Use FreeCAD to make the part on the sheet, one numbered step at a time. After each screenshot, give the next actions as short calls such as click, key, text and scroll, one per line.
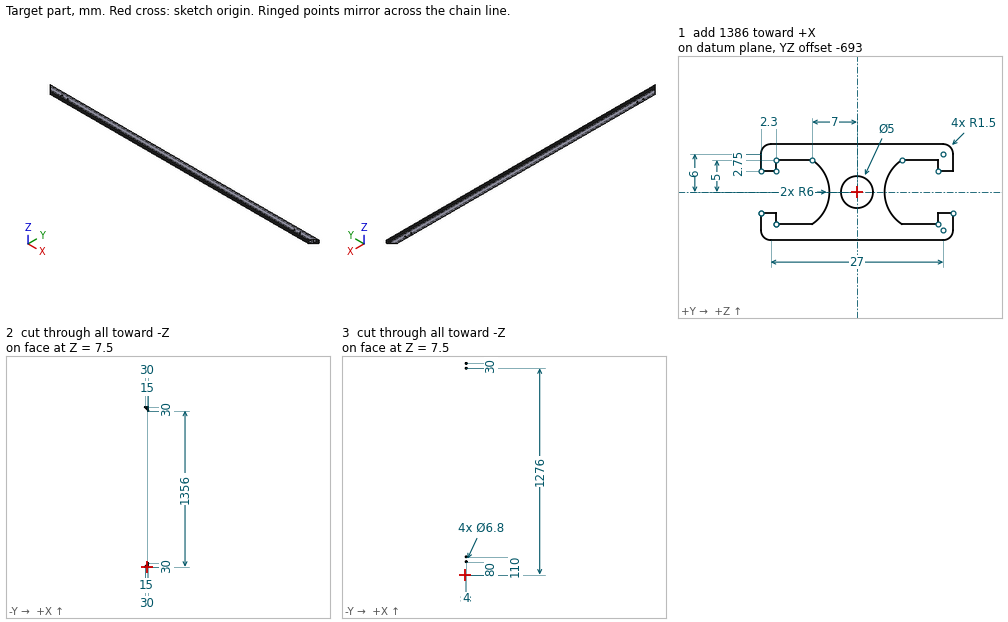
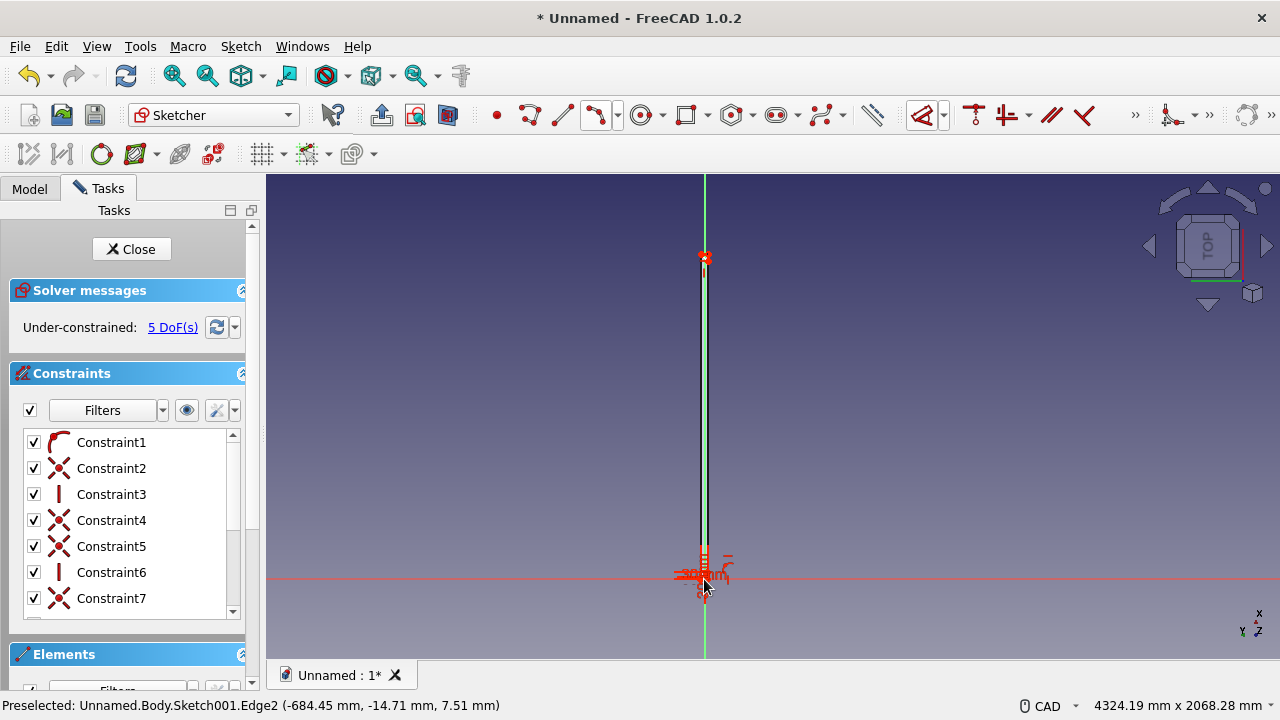
scroll(708, 260, up, 12)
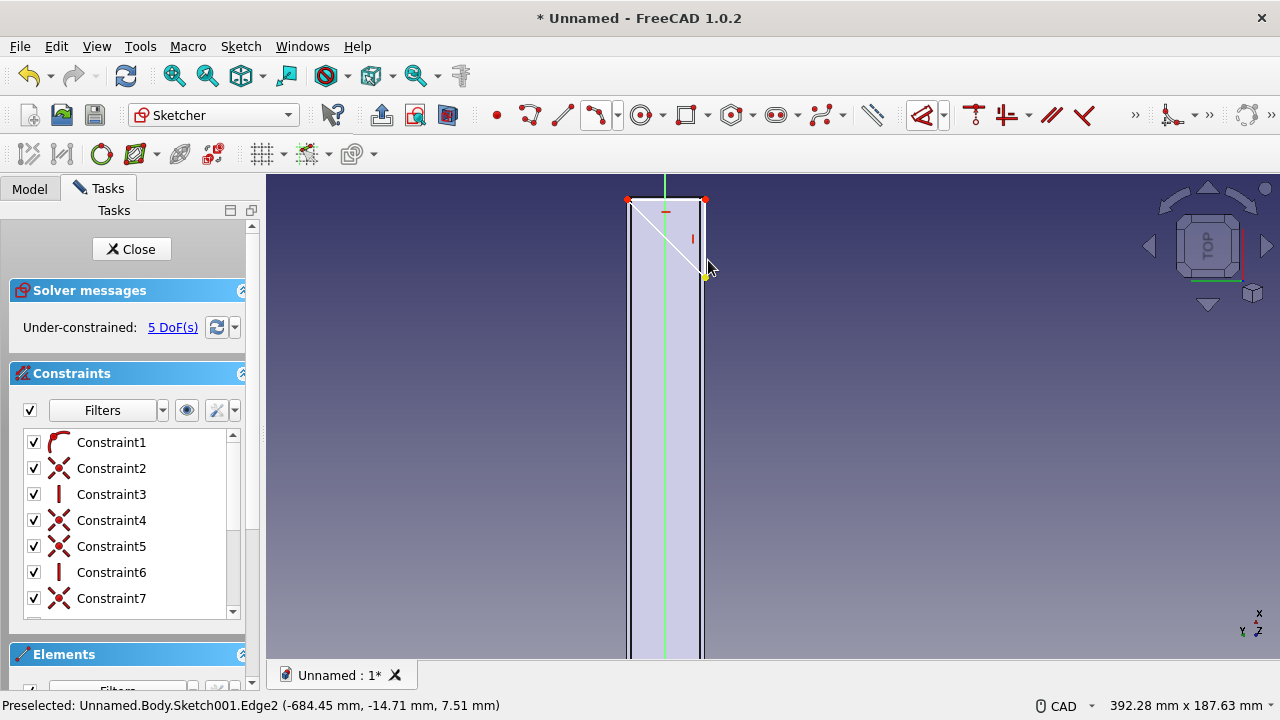
click(705, 254)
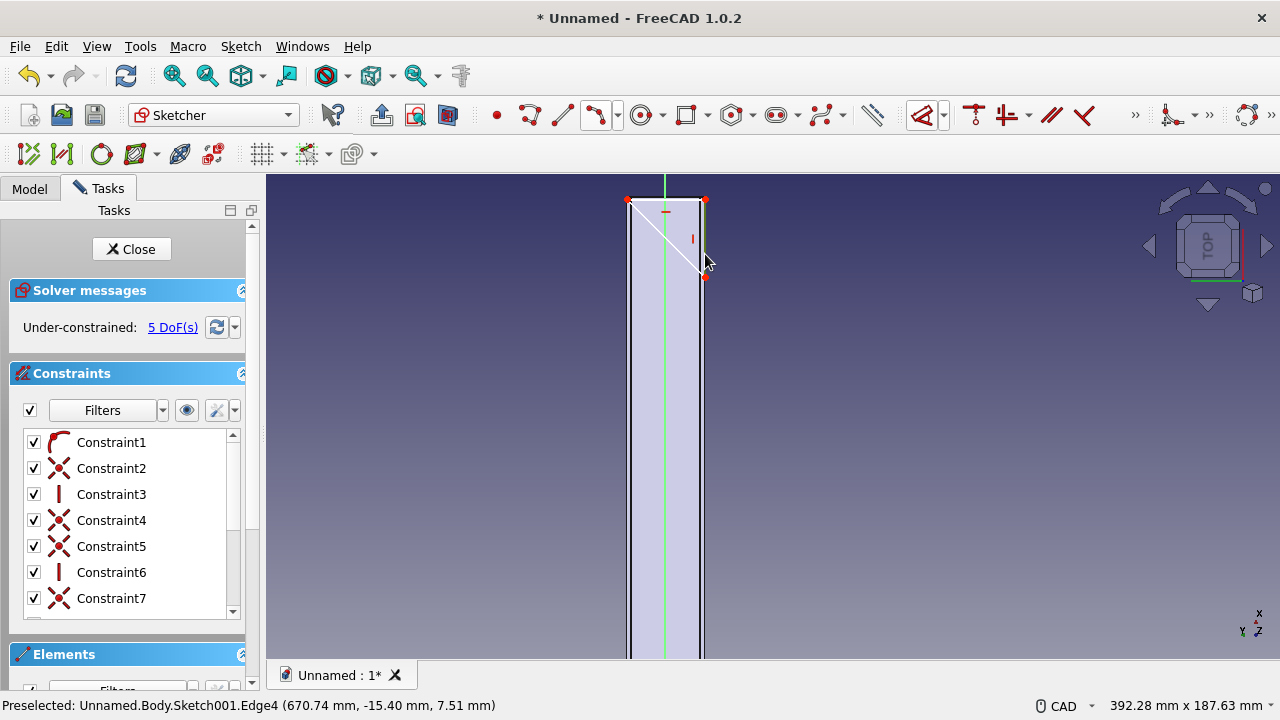
key(i)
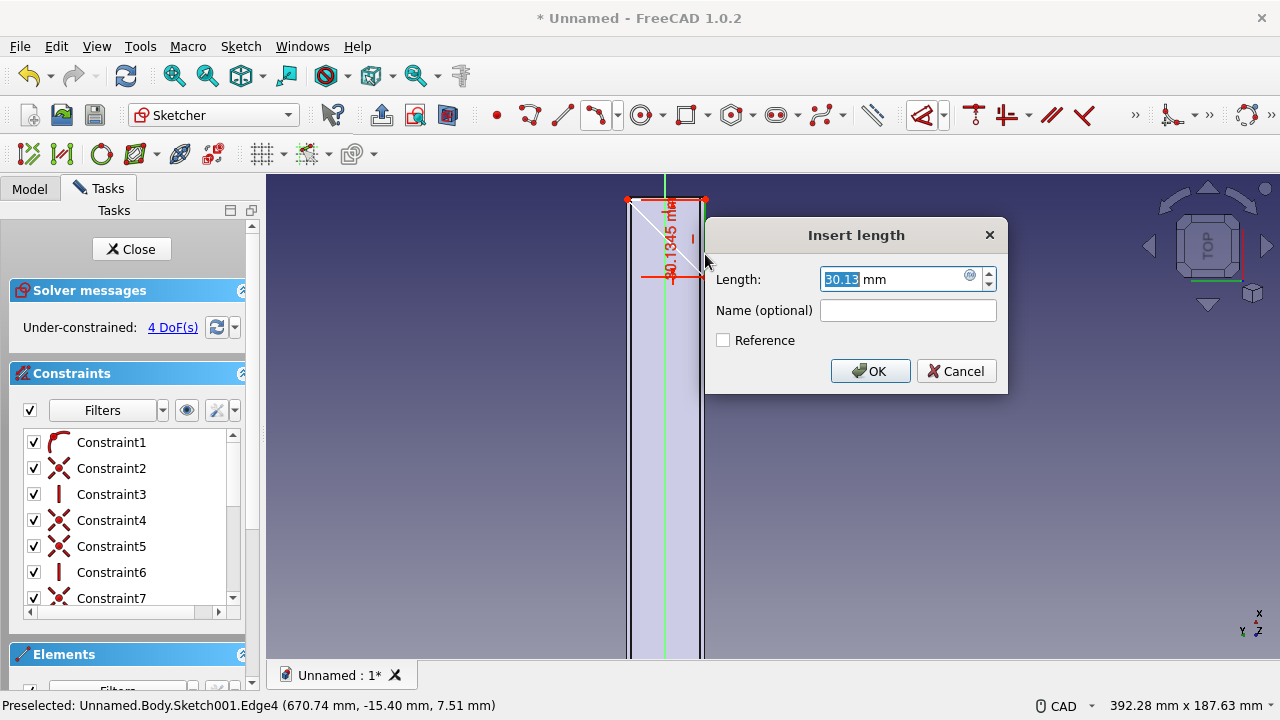
text(30)
key(Return)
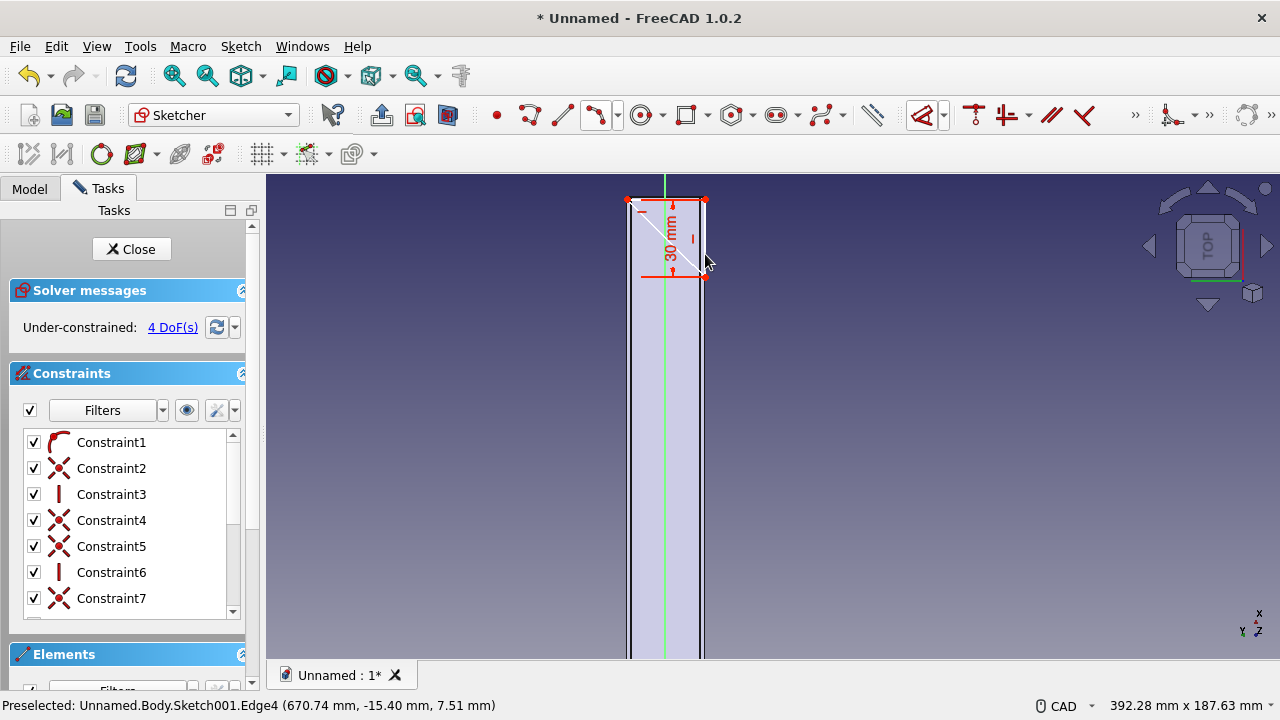
scroll(708, 260, down, 12)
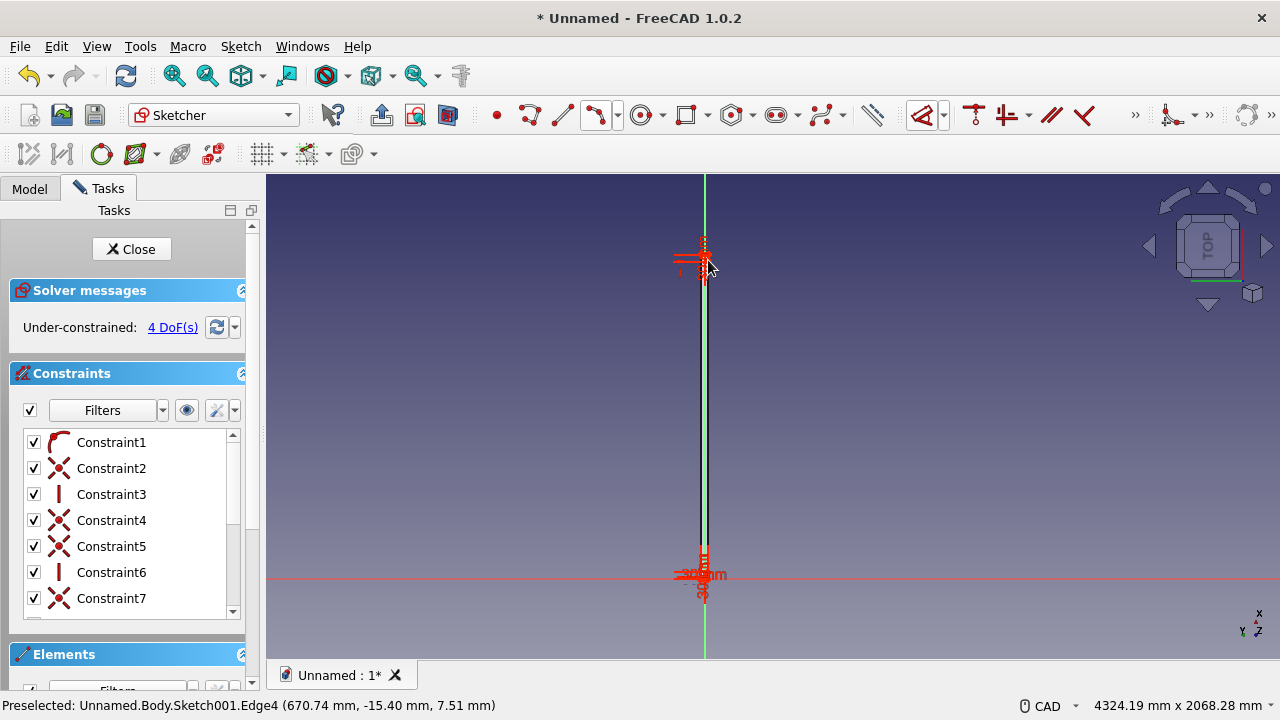
scroll(706, 255, up, 12)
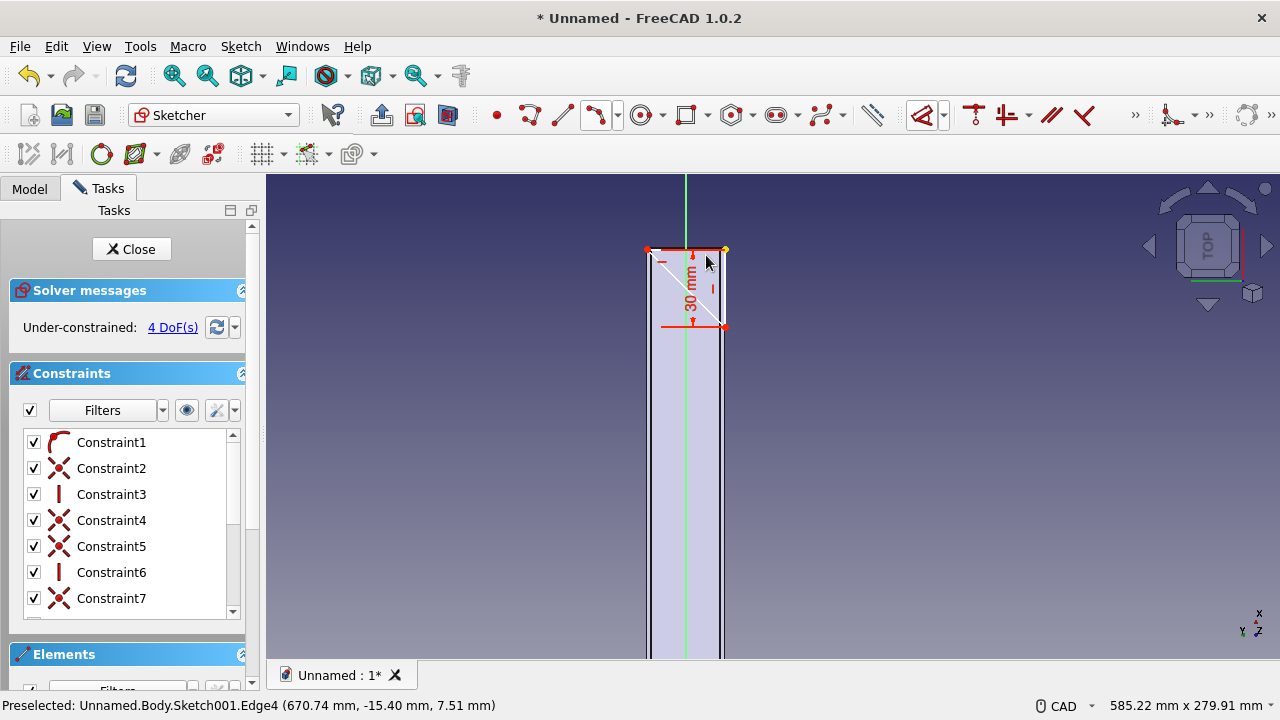
click(702, 250)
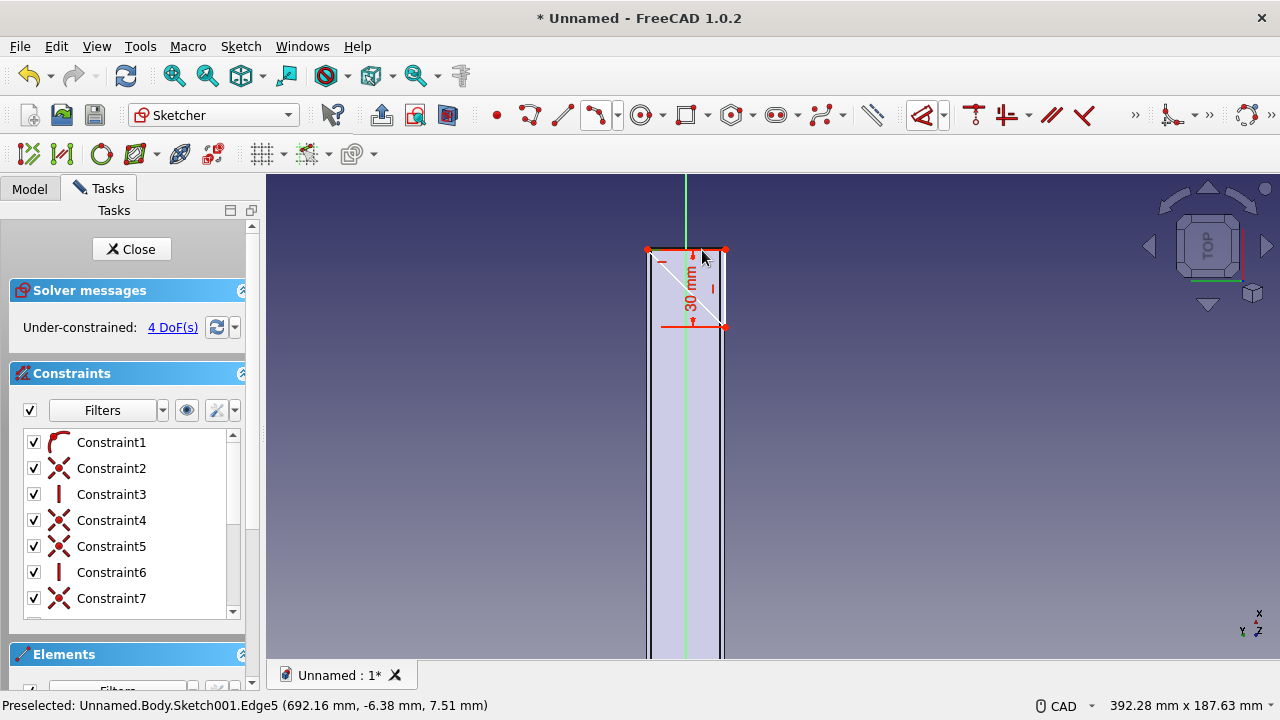
key(l)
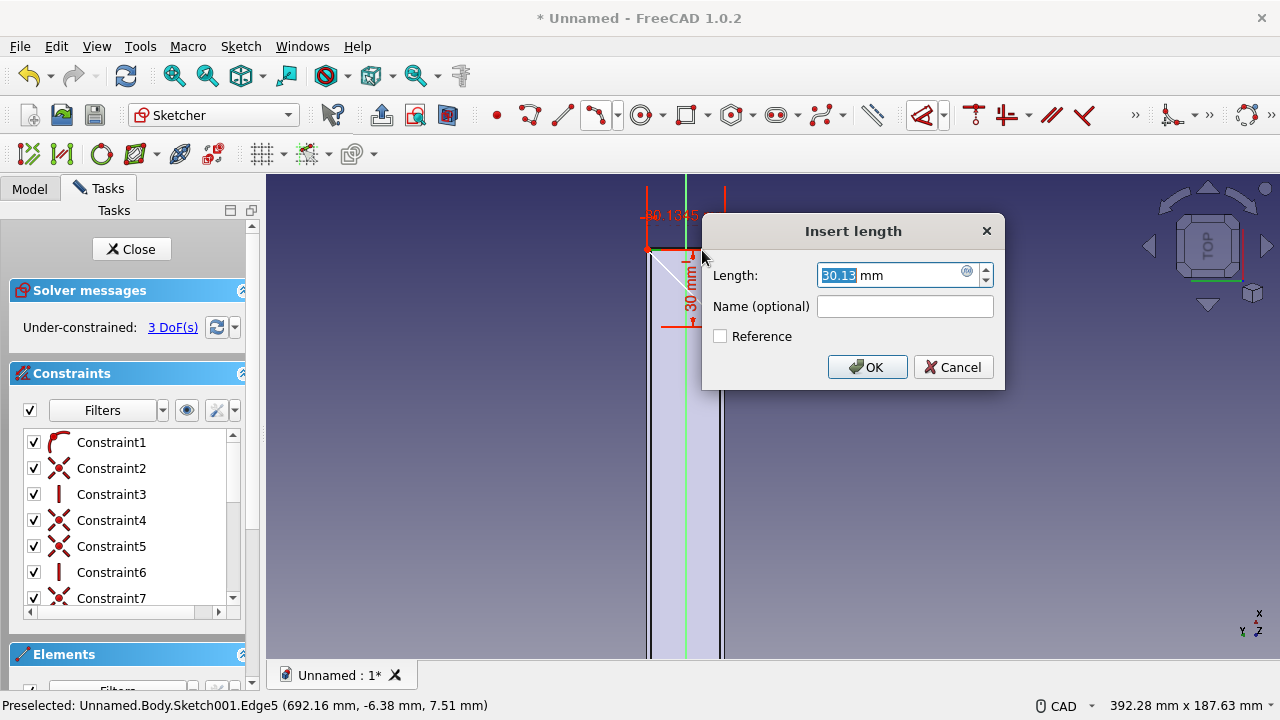
text(30)
key(Return)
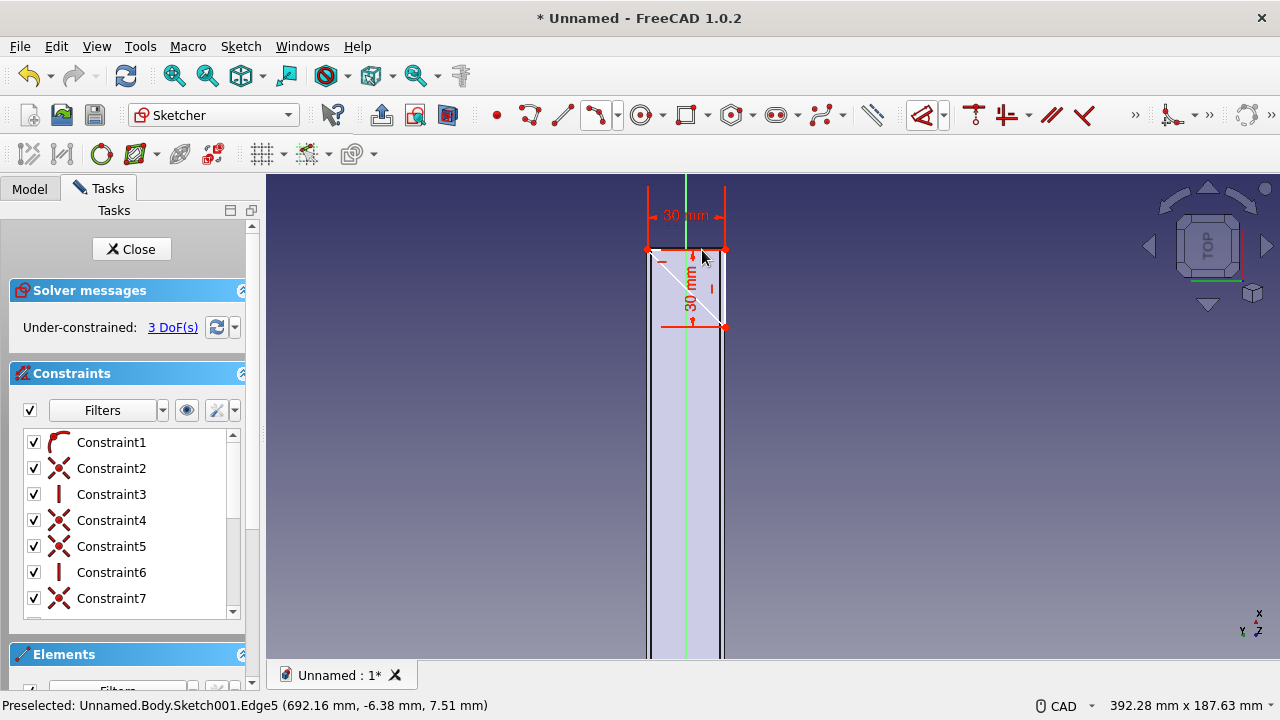
scroll(706, 255, down, 12)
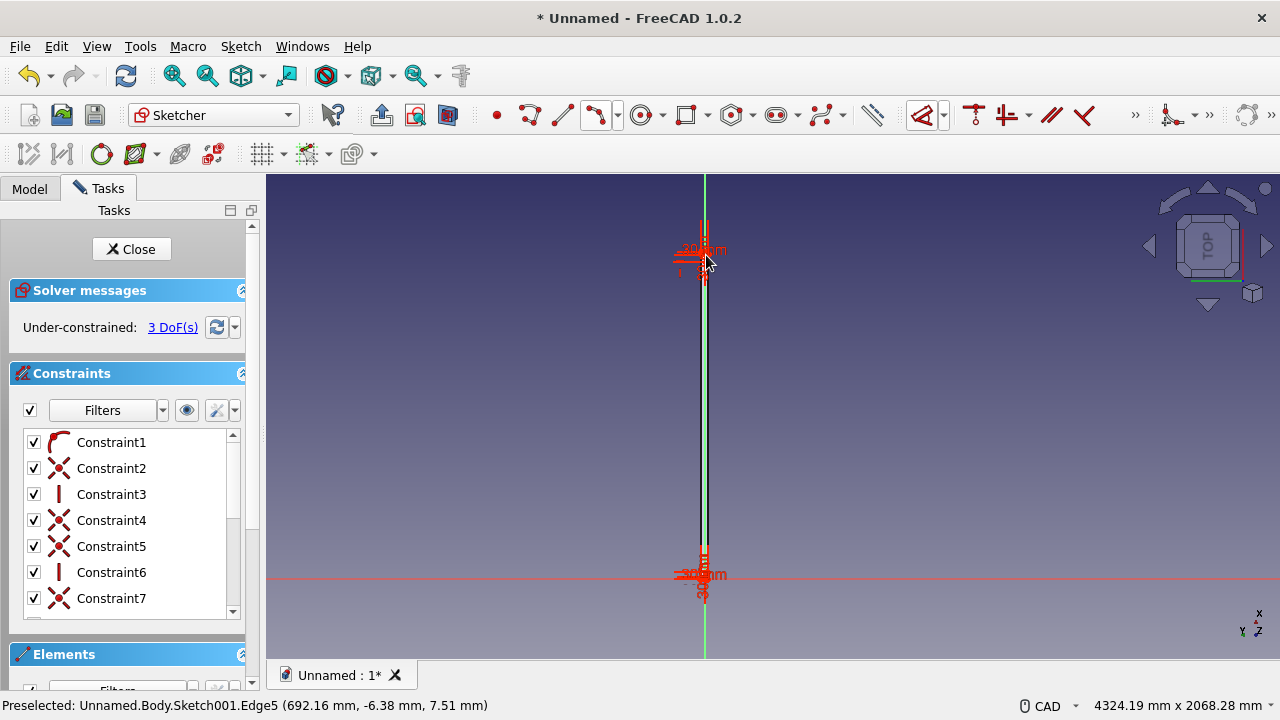
scroll(701, 579, up, 13)